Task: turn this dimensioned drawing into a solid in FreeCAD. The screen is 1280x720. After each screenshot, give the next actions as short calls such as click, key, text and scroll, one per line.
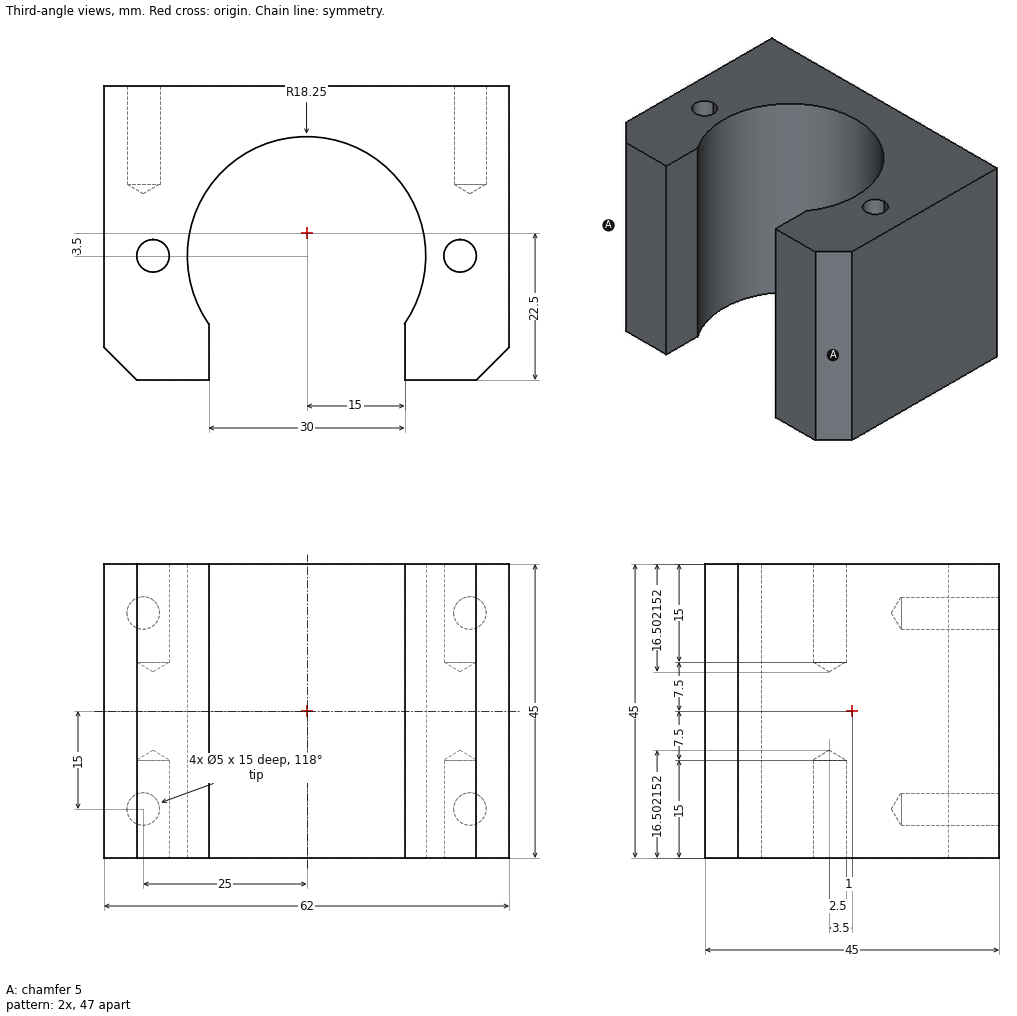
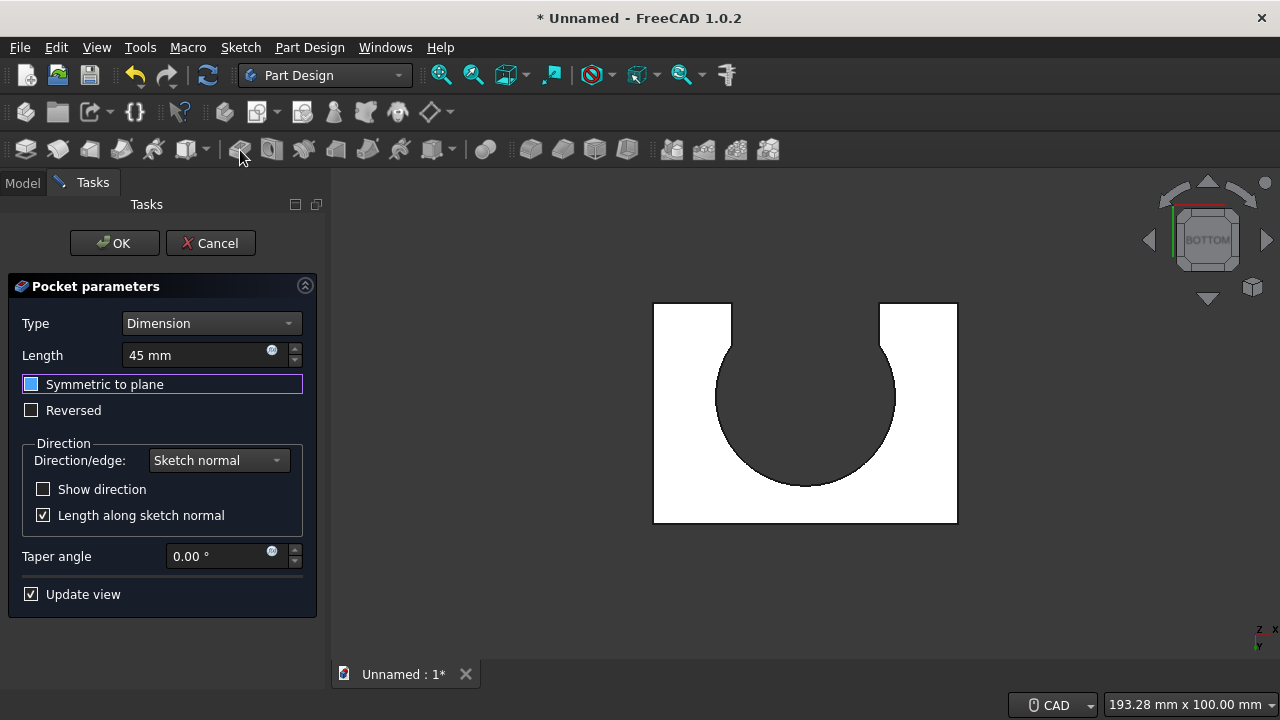
click(115, 243)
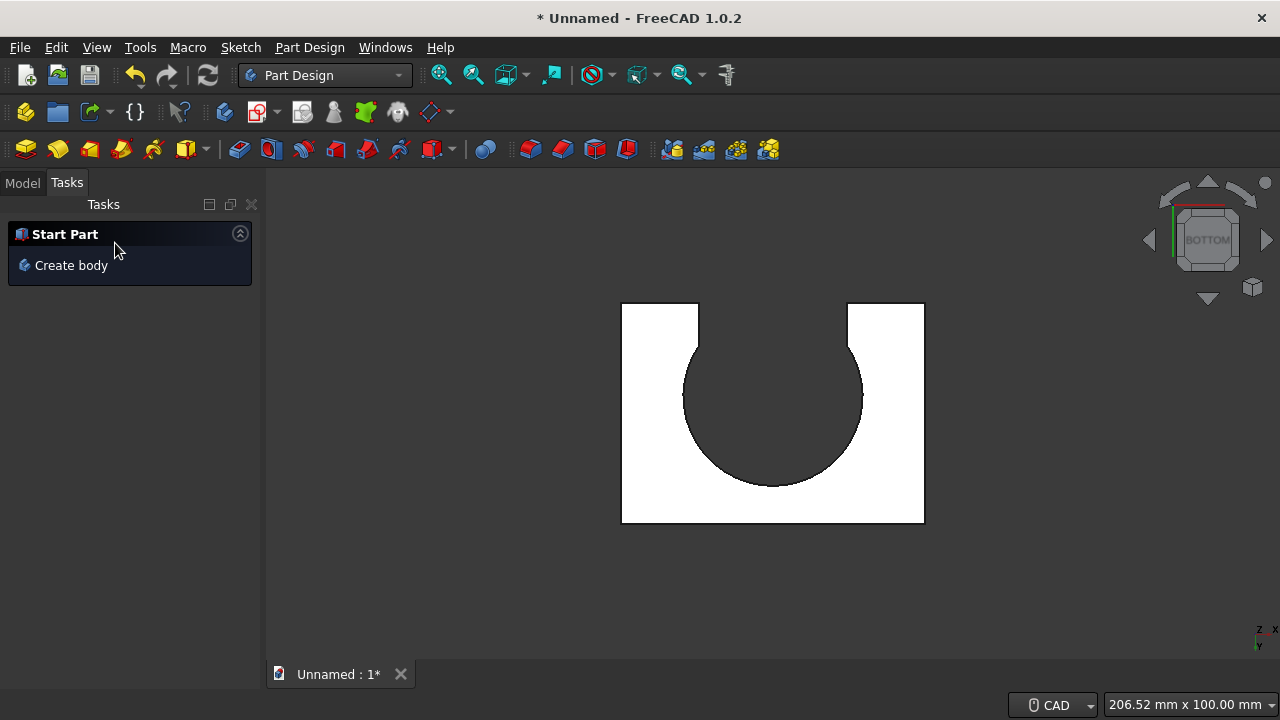
key(0)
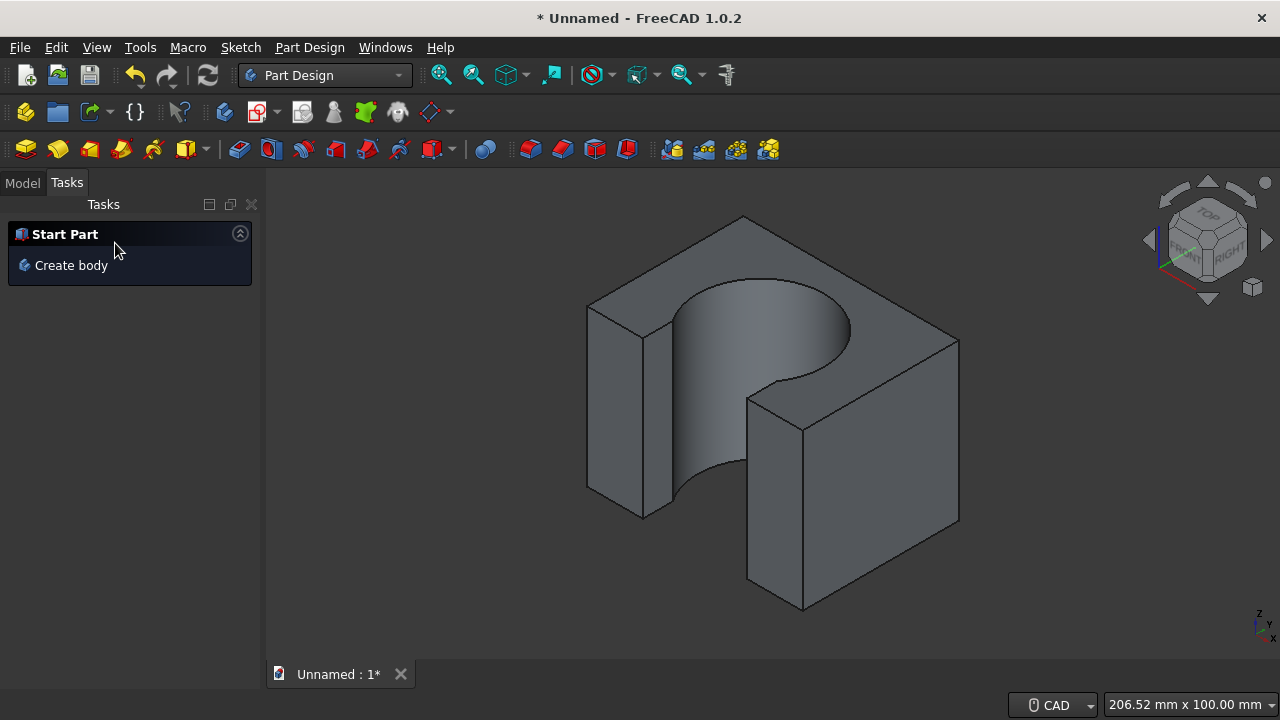
click(803, 520)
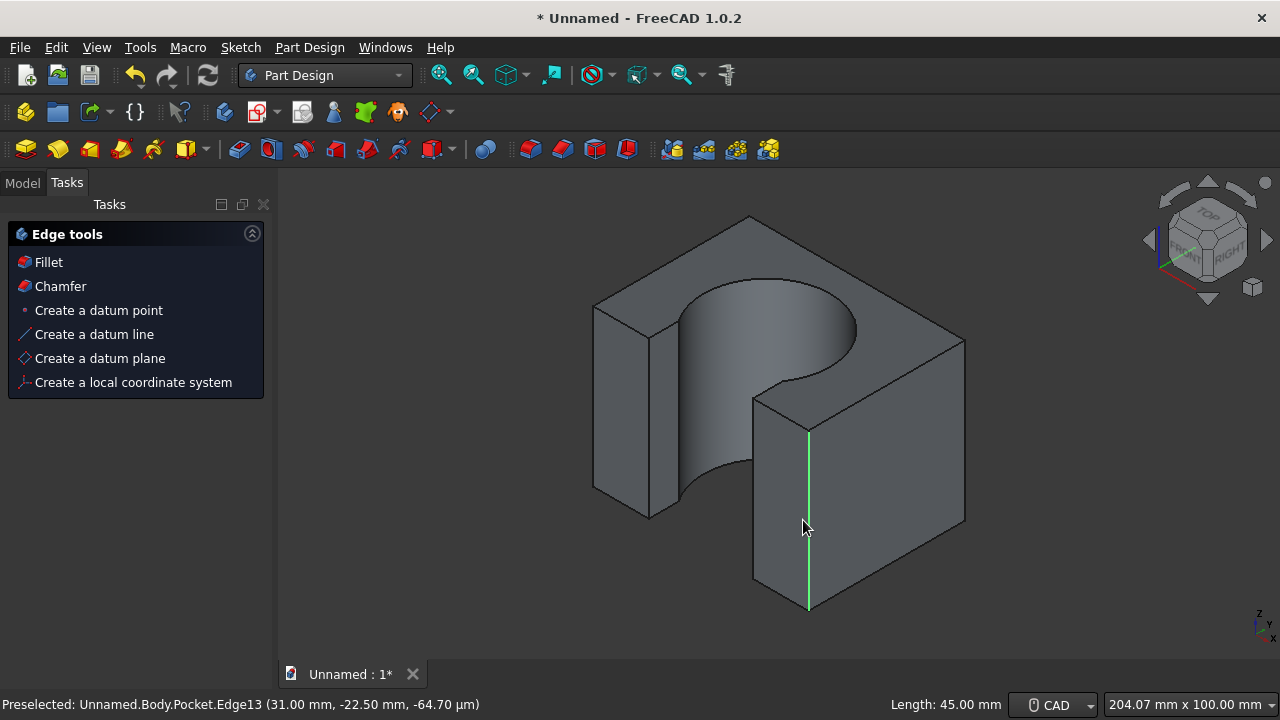
key(2)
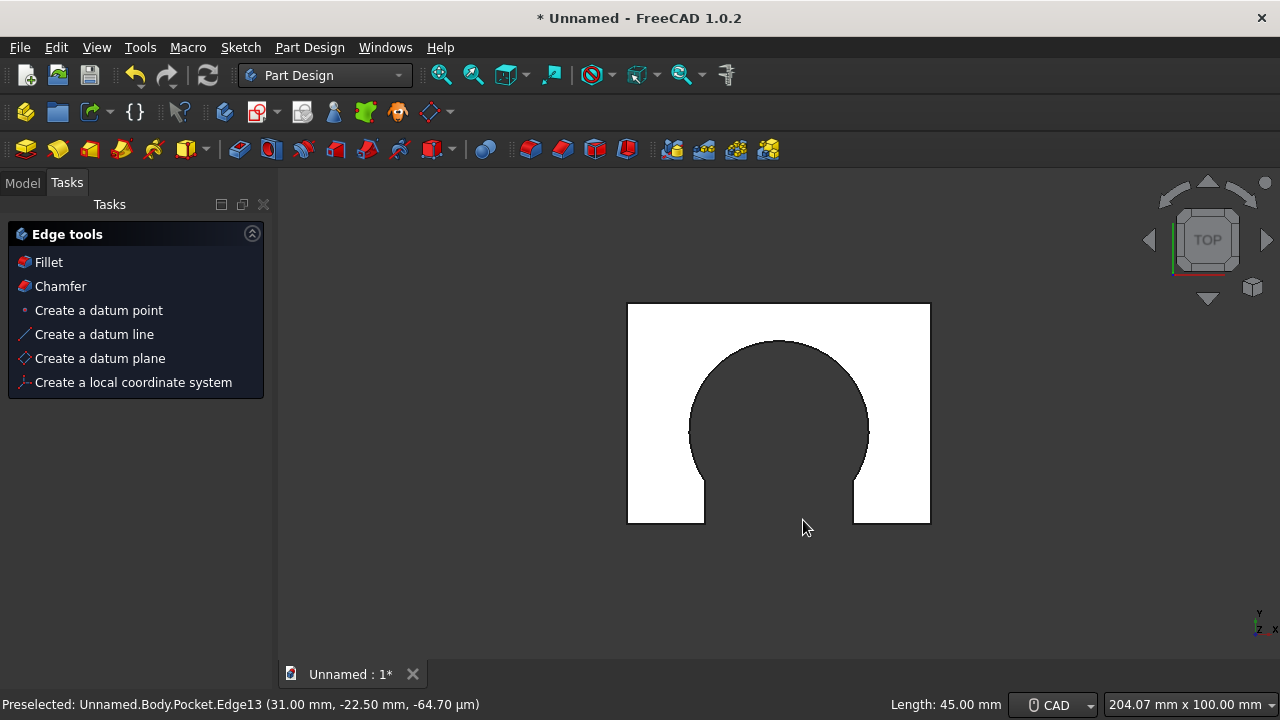
key(1)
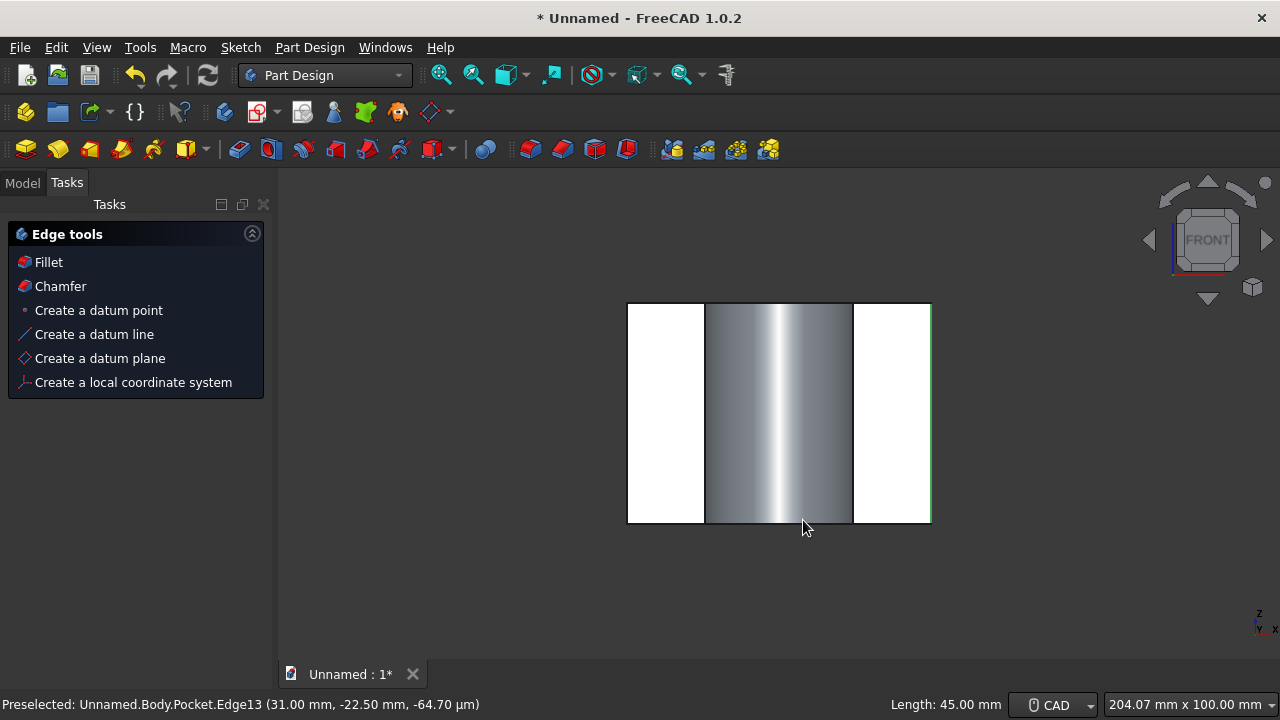
click(627, 412, ctrl)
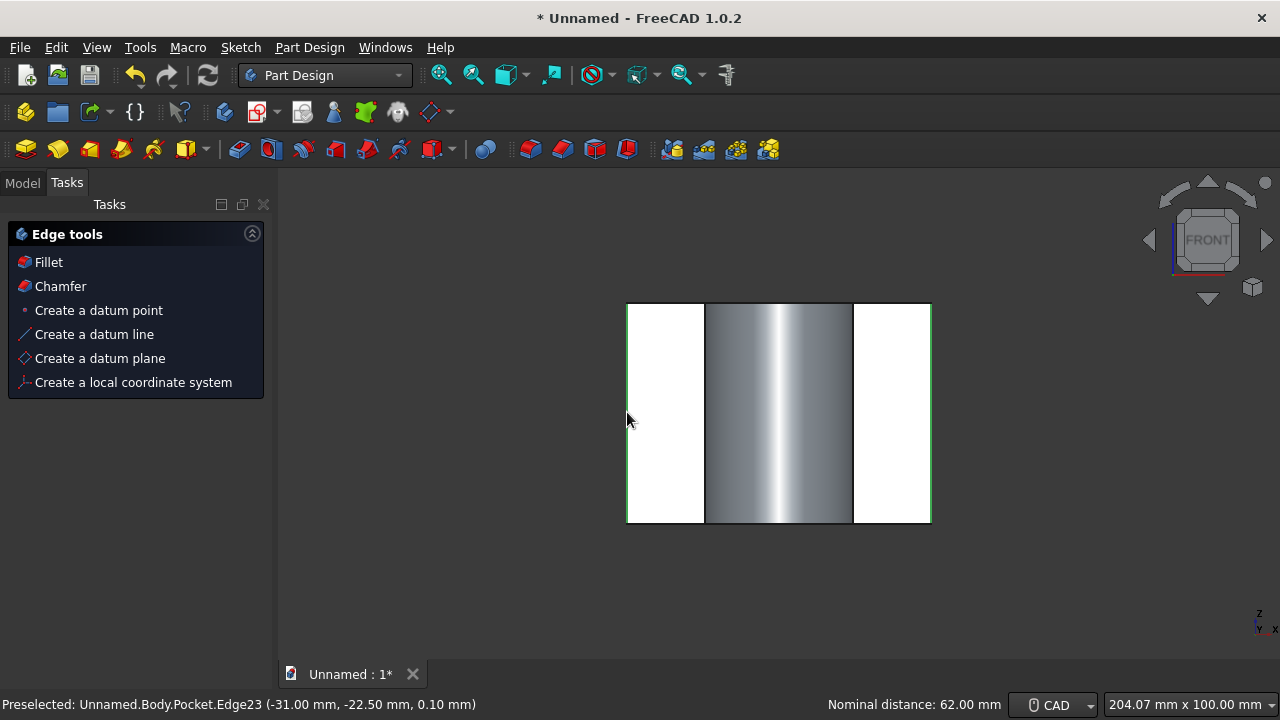
click(564, 150)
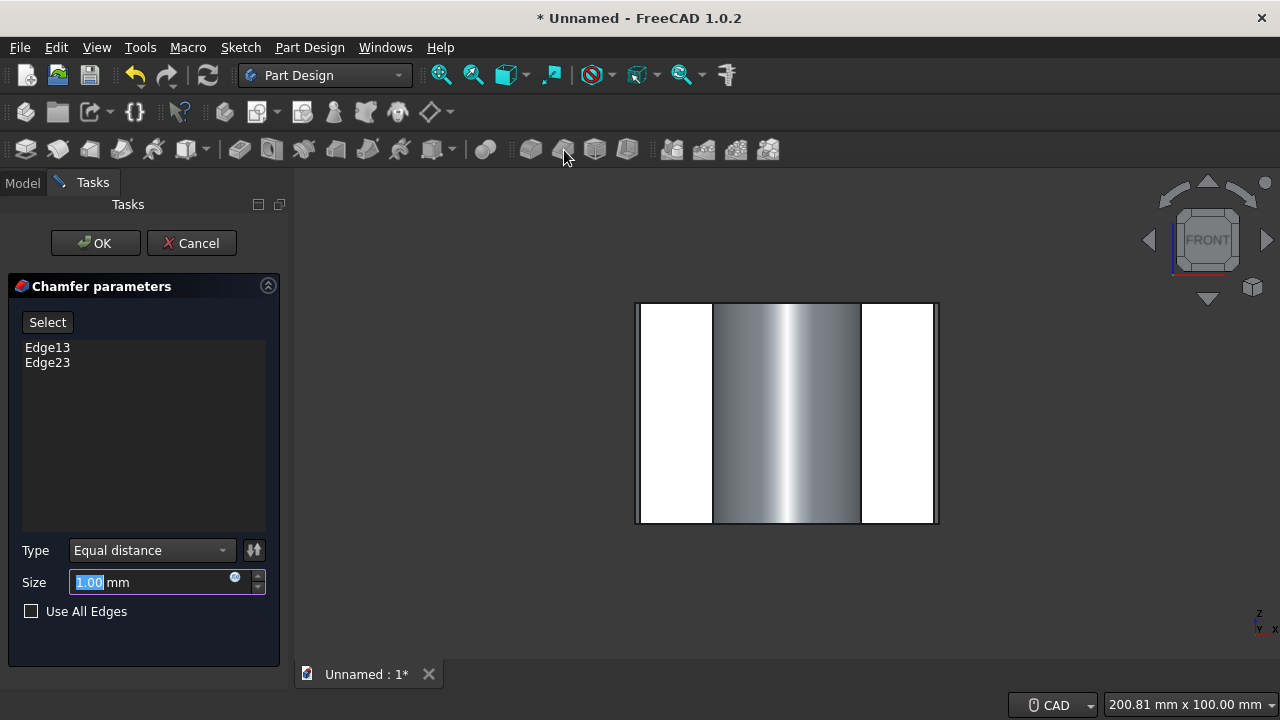
text(5)
key(Tab)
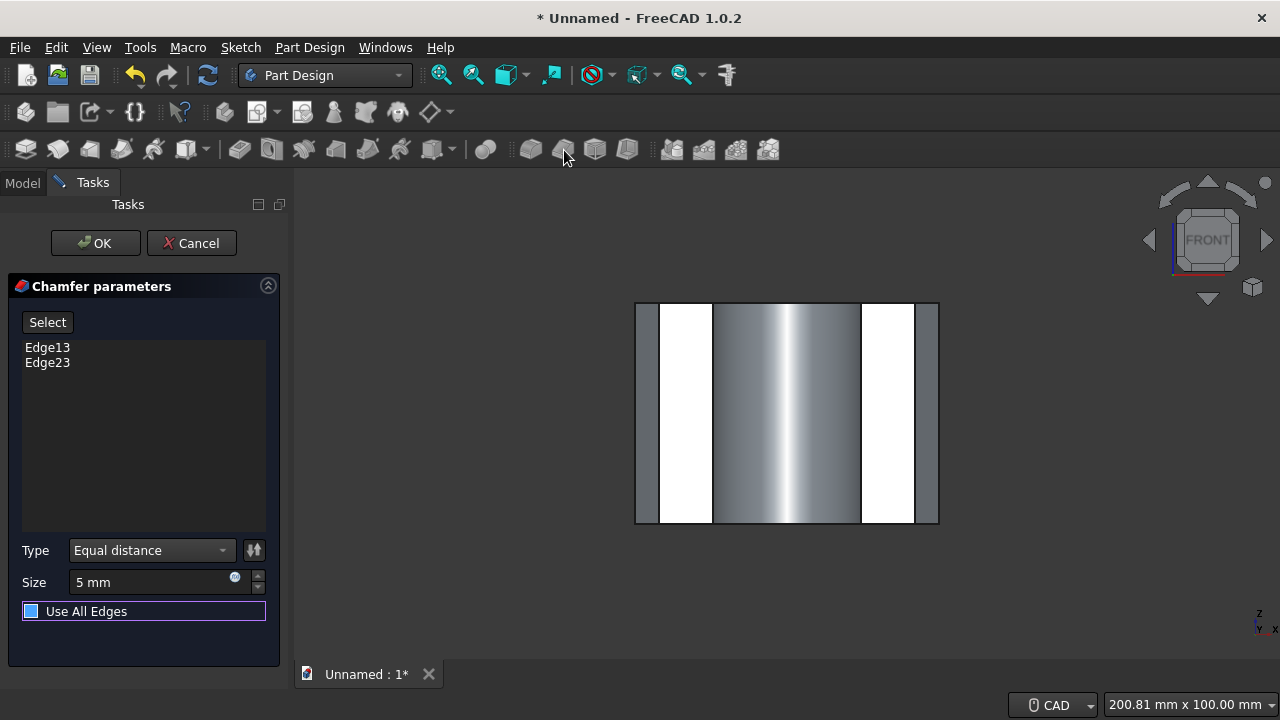
click(96, 243)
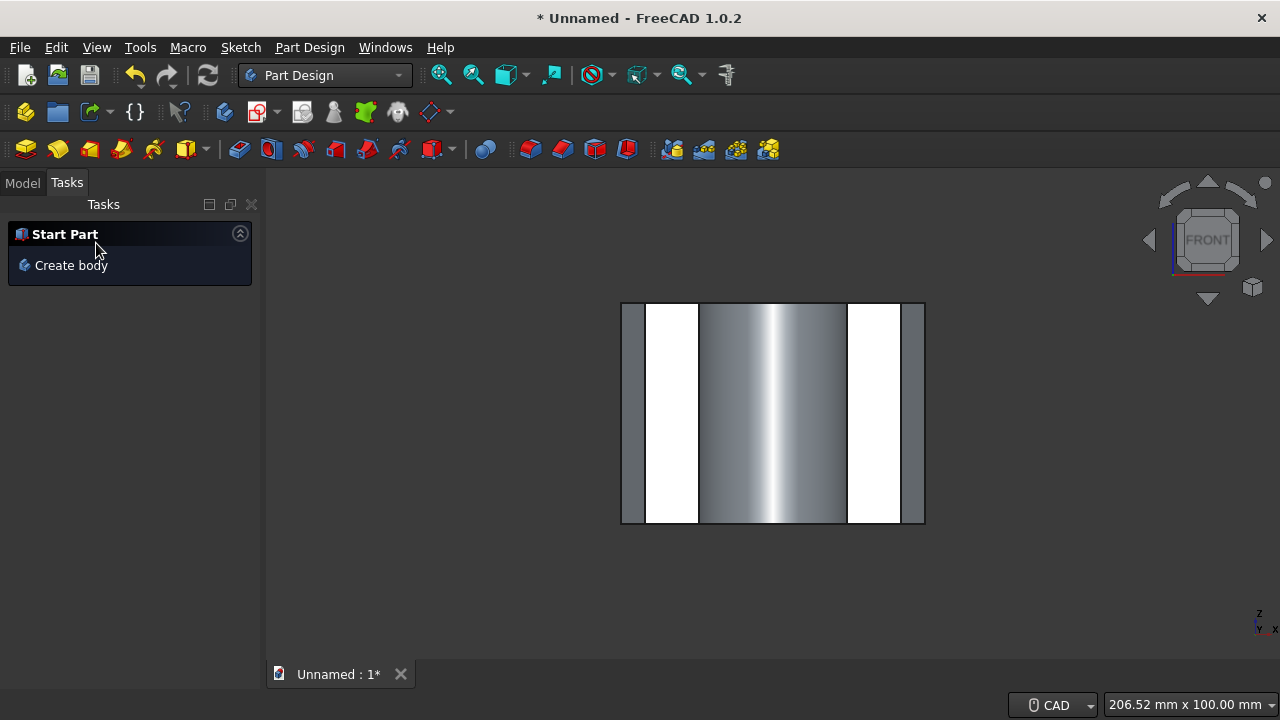
key(4)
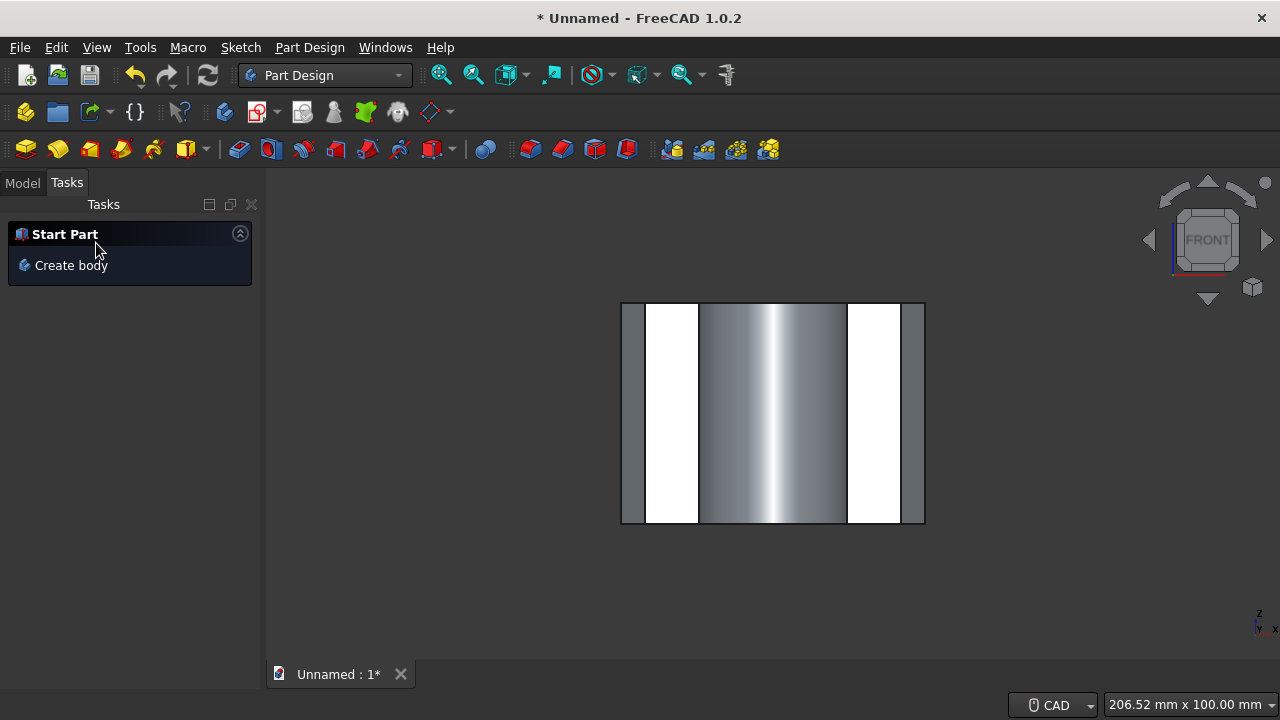
click(773, 412)